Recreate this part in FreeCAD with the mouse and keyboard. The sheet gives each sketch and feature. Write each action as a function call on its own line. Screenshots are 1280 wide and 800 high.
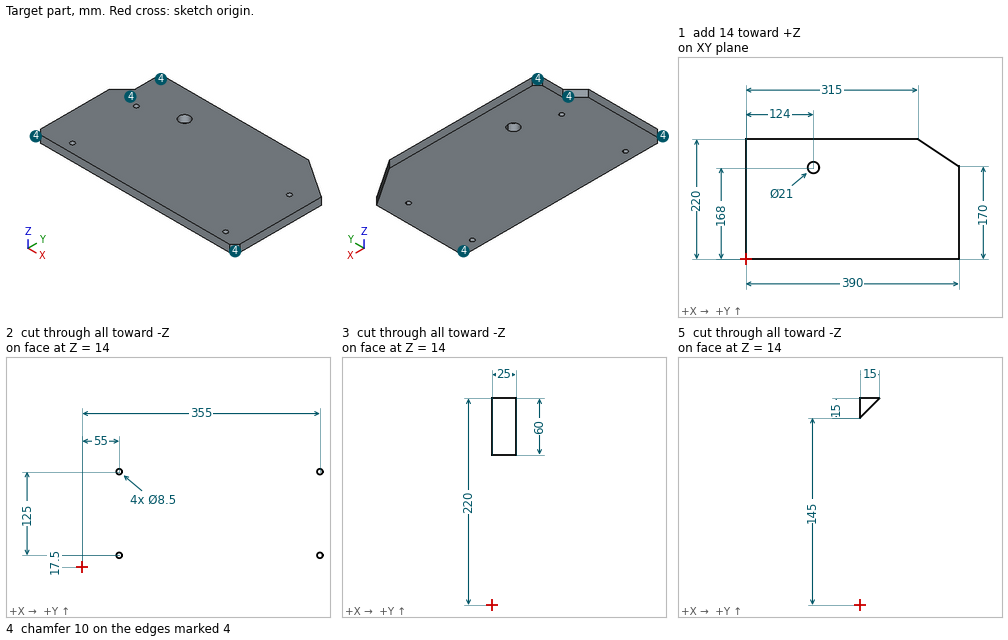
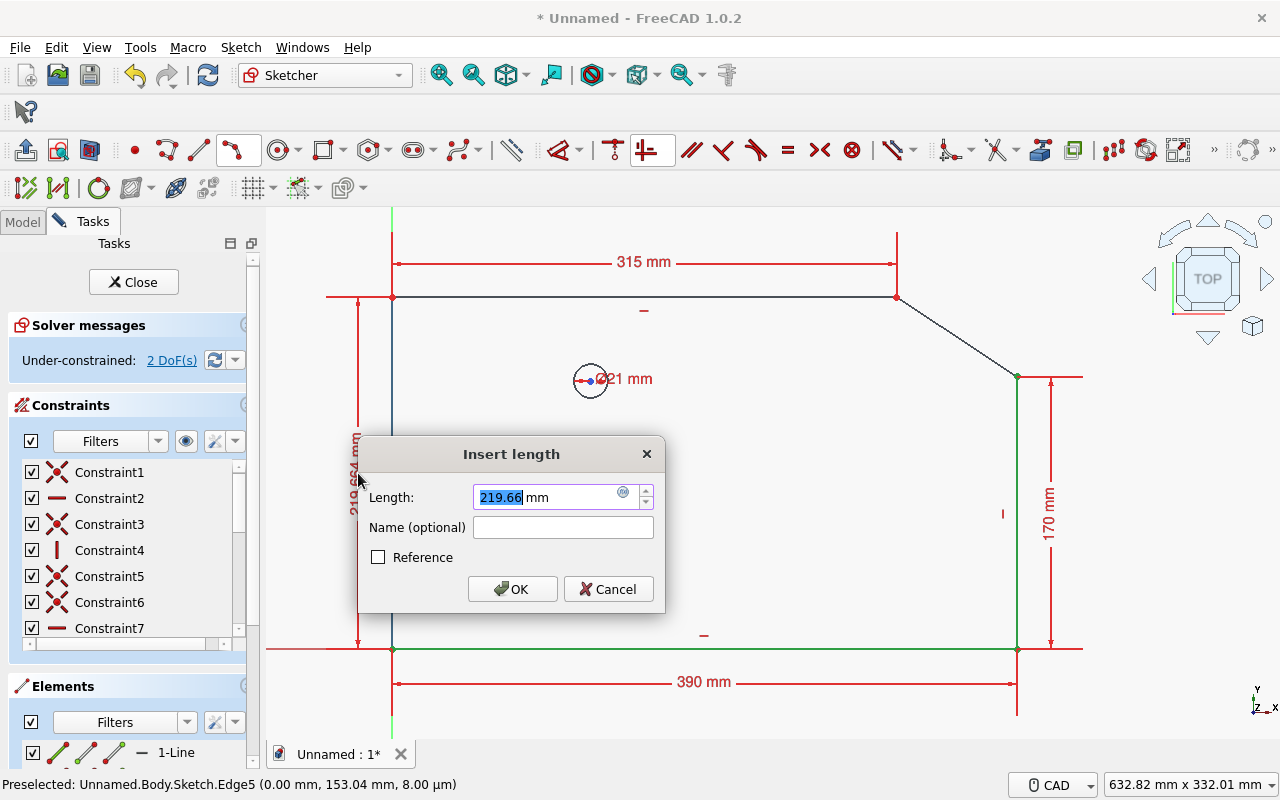
text(220)
key(Return)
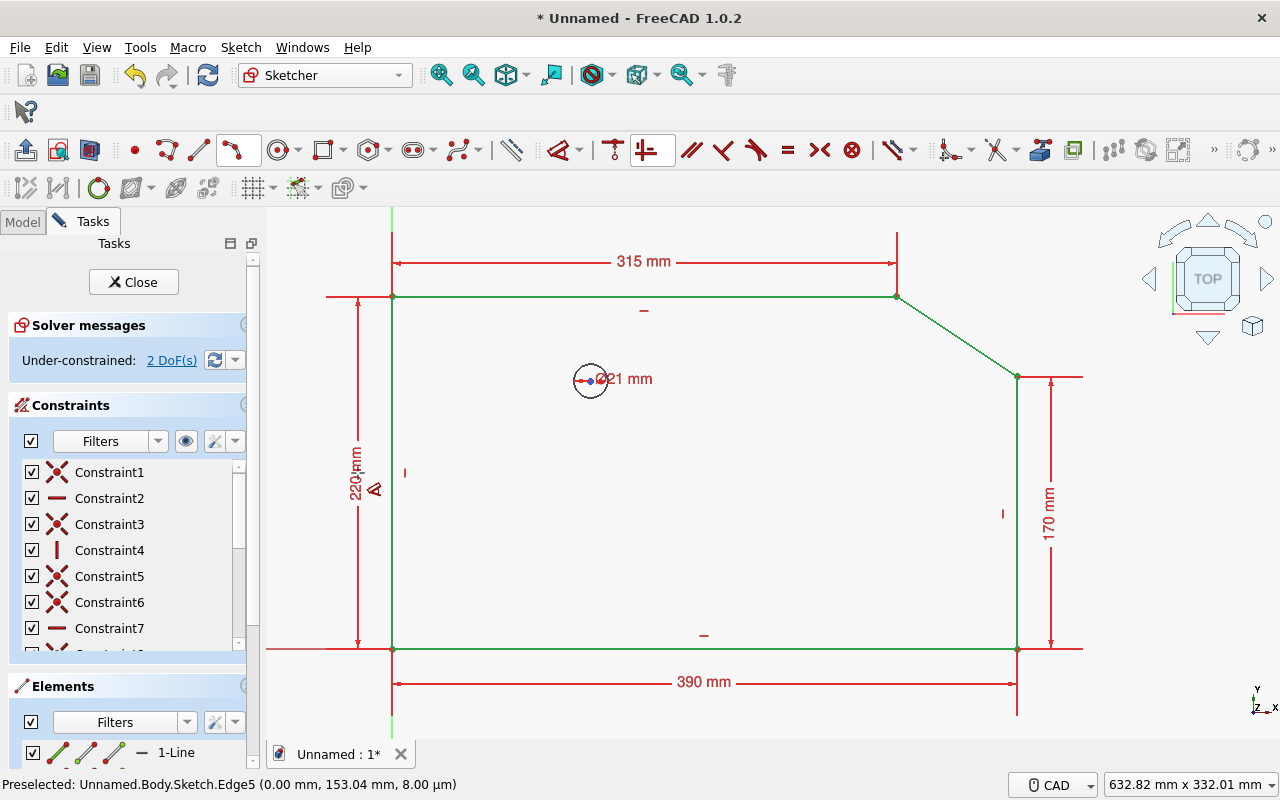
click(591, 381)
click(492, 683)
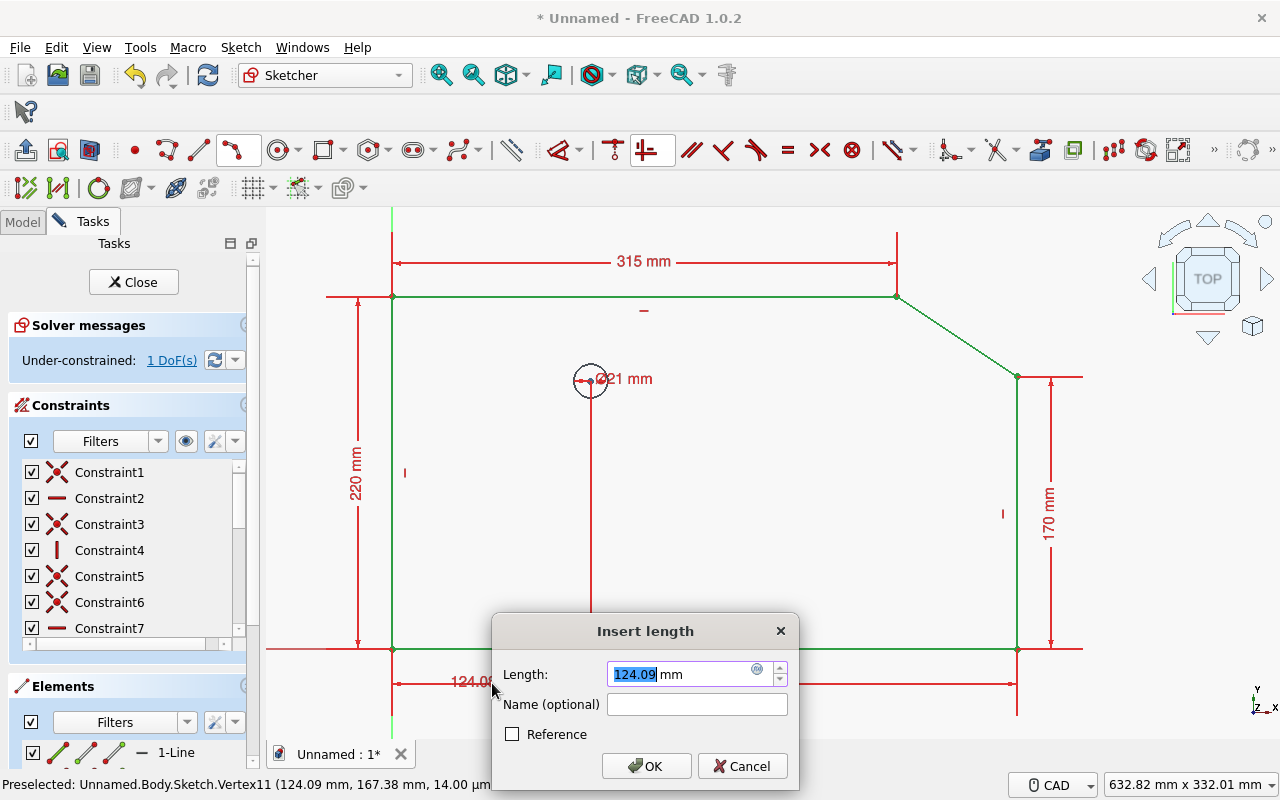
text(124)
key(Return)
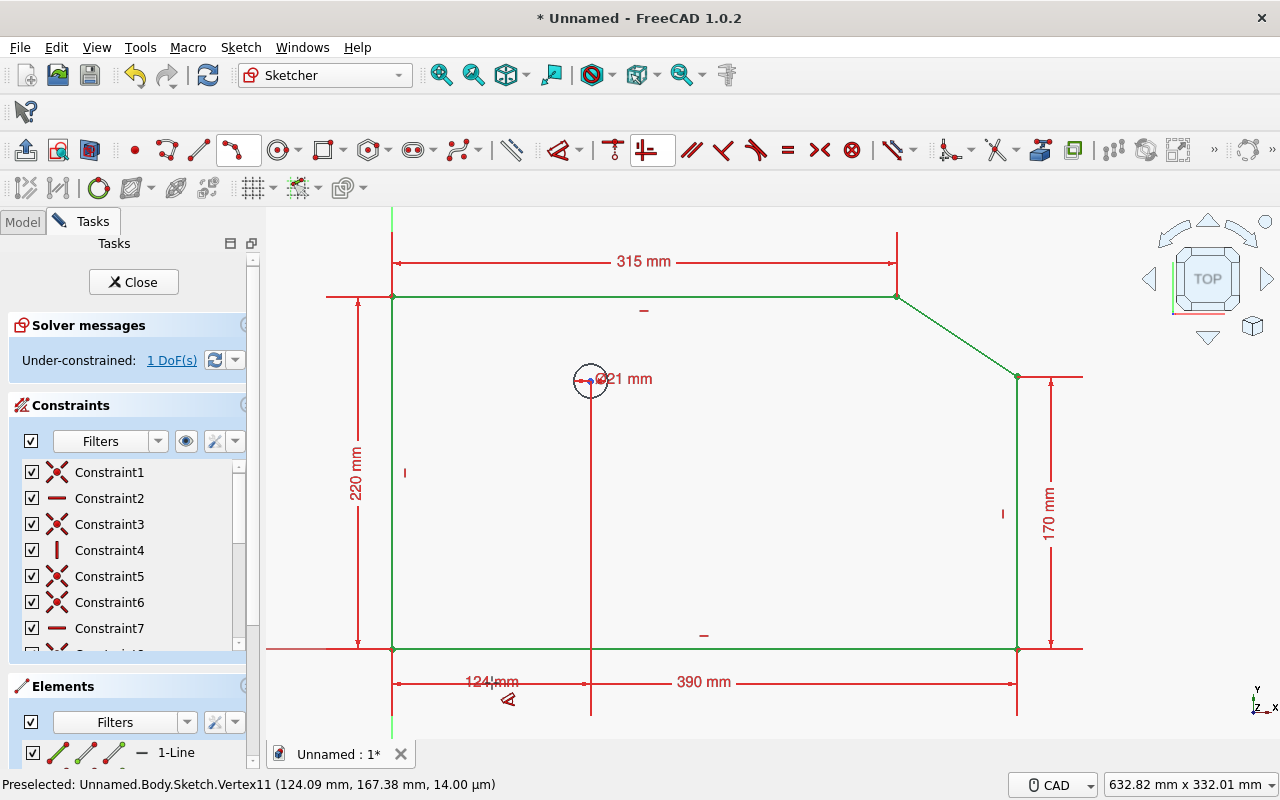
click(591, 381)
click(358, 515)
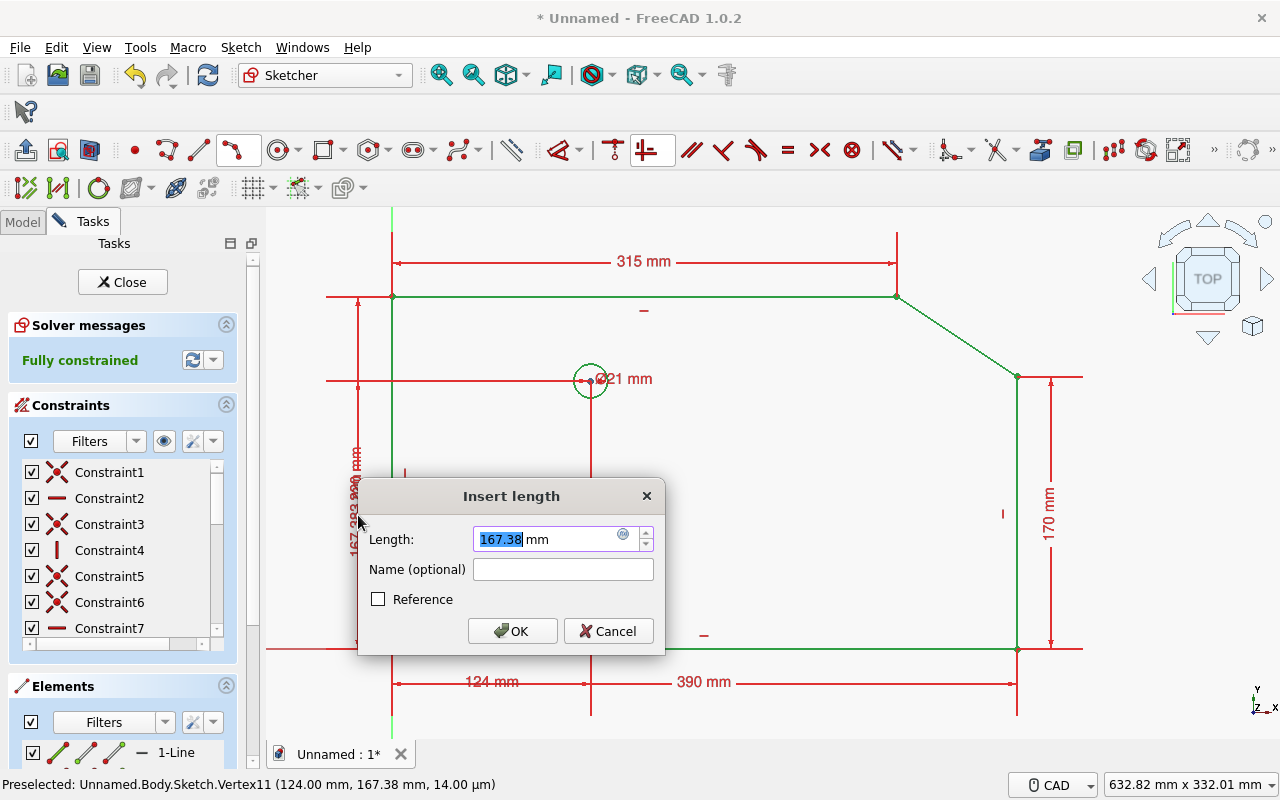
text(168)
key(Return)
key(Escape)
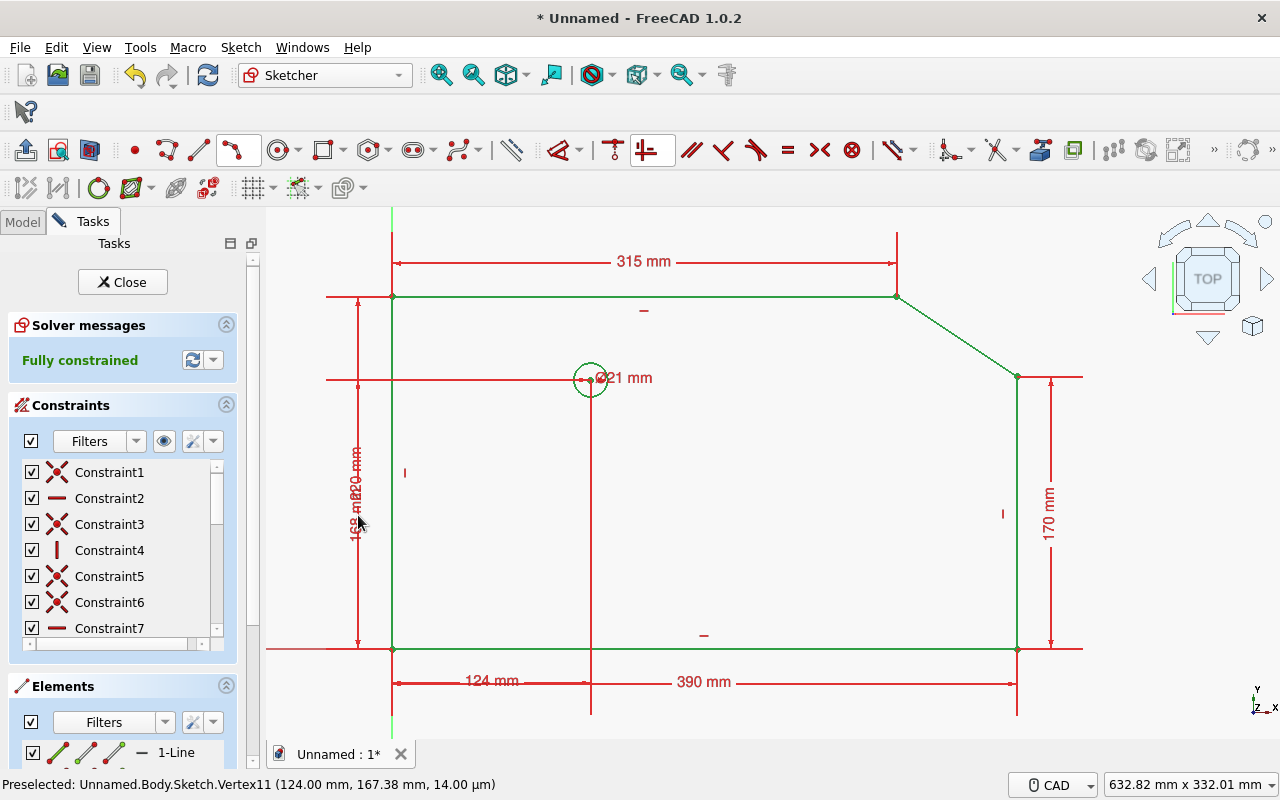
click(123, 282)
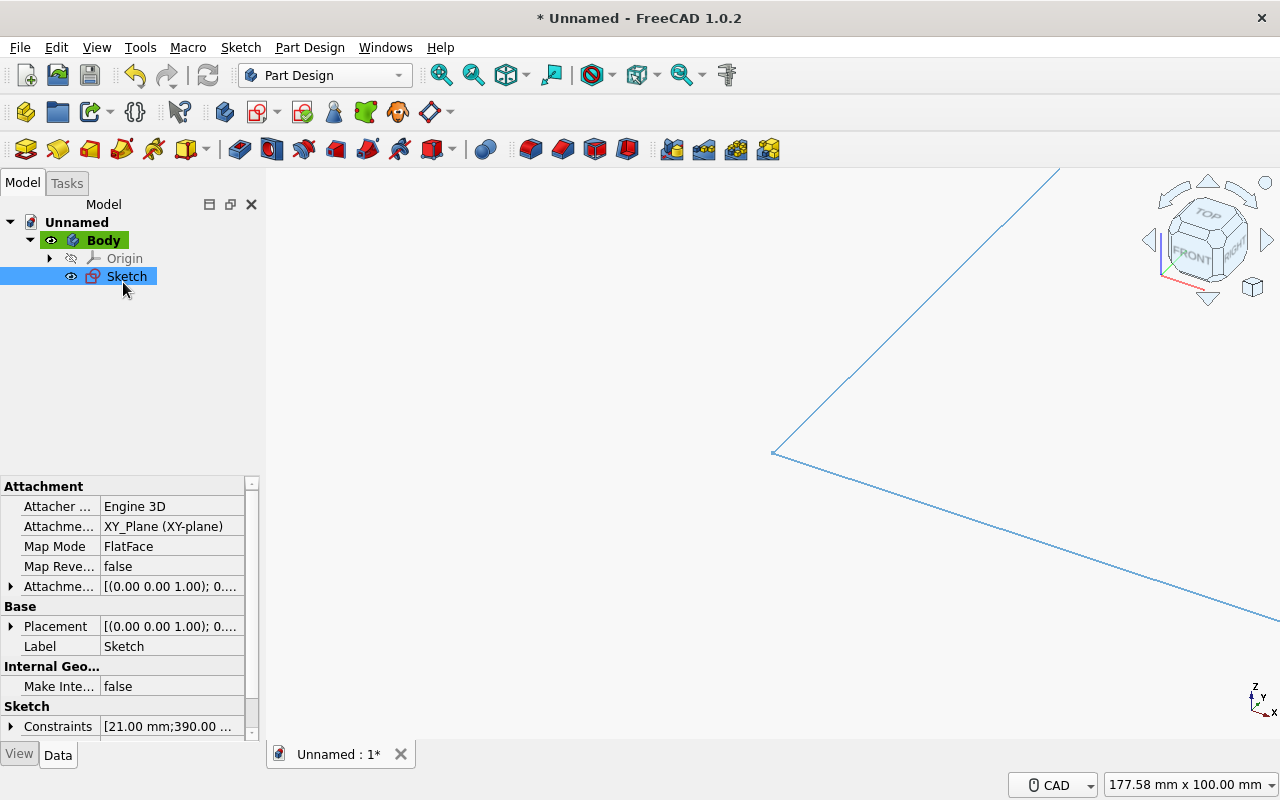
click(26, 150)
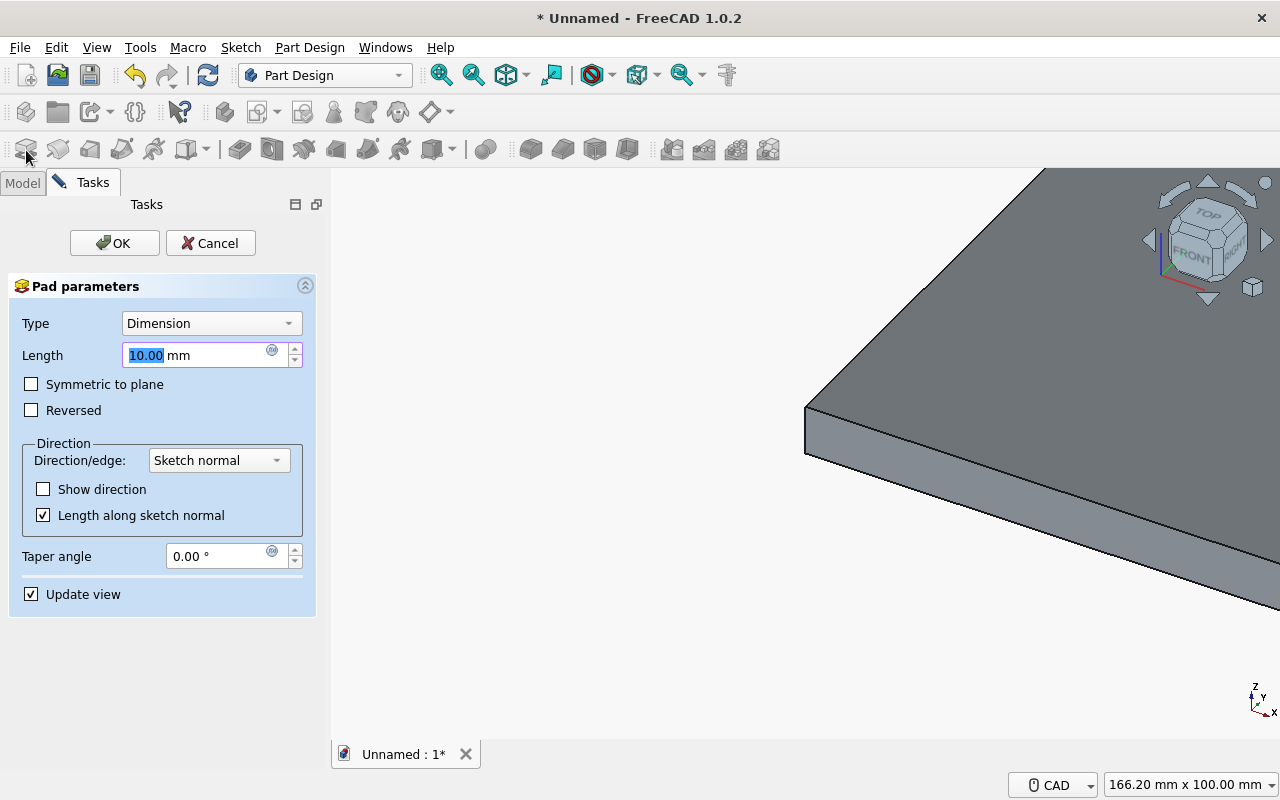
text(14)
key(Tab)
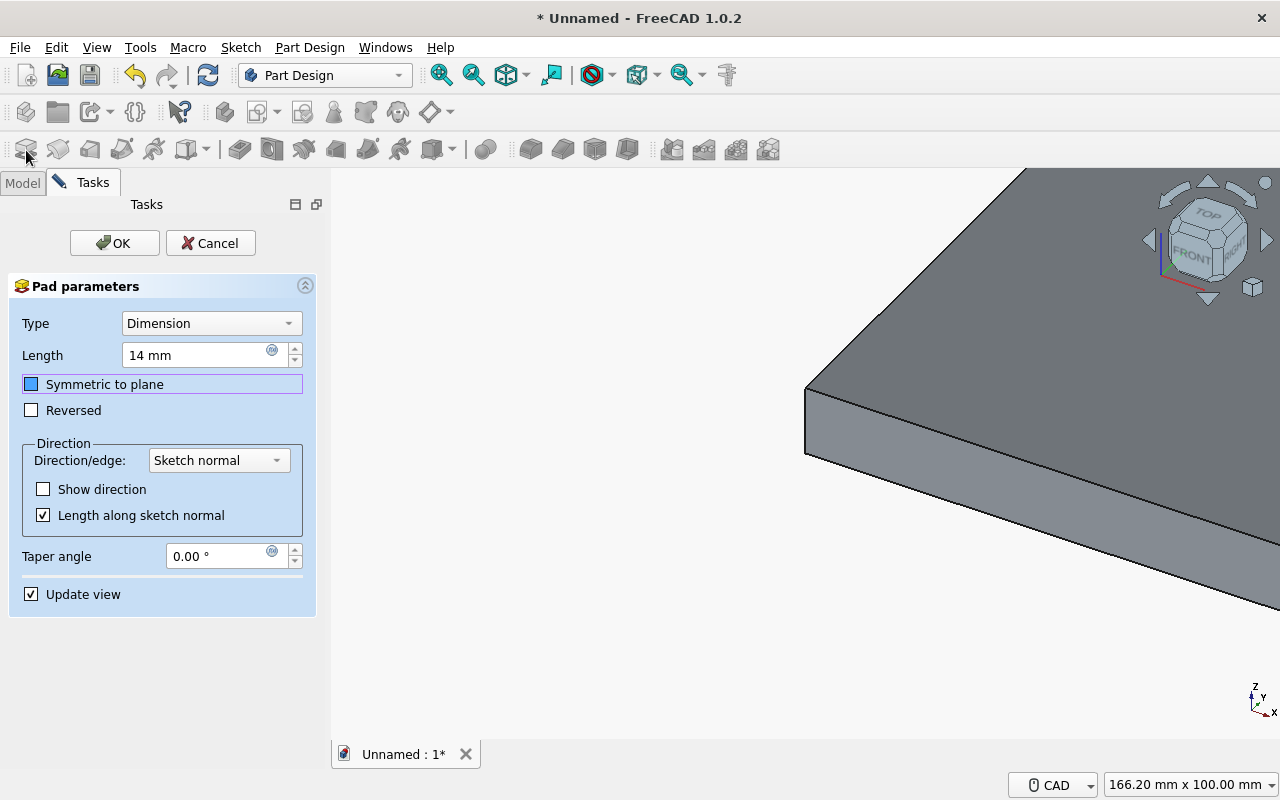
click(115, 243)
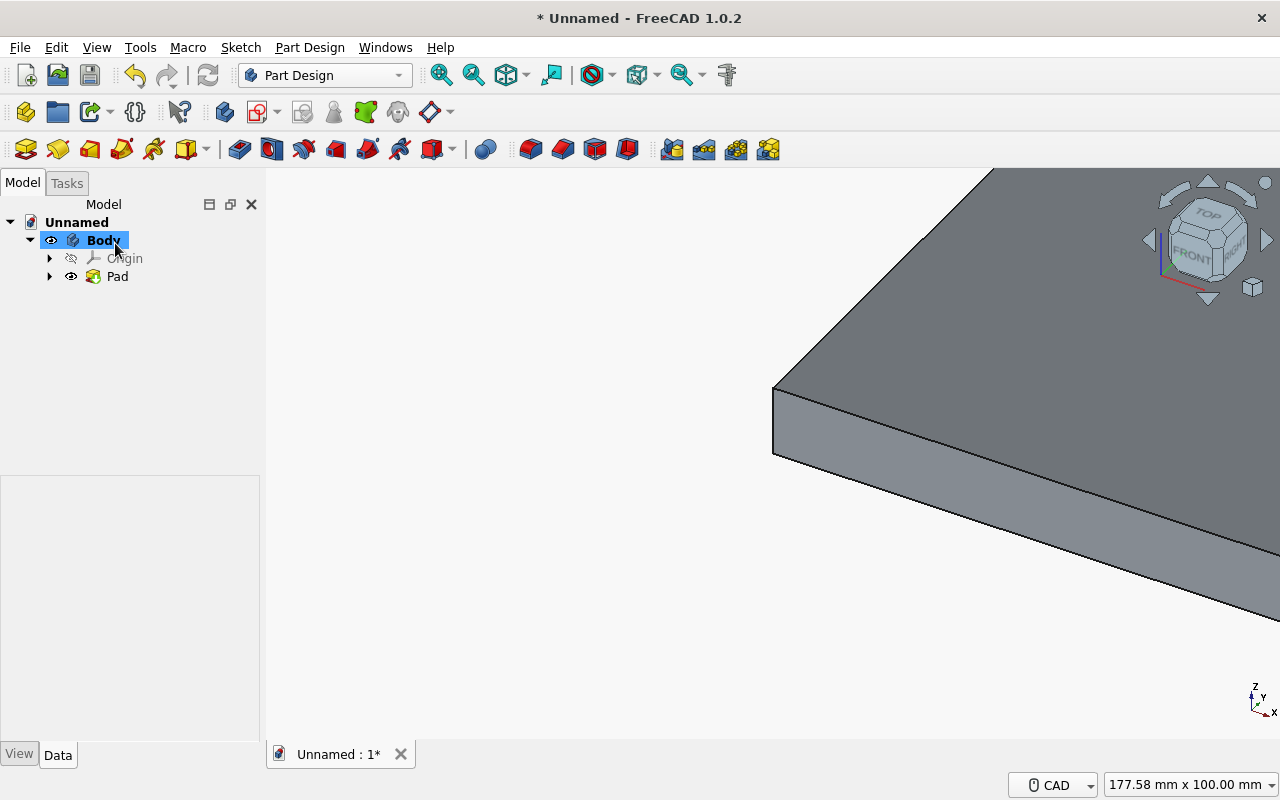
key(v)
key(f)